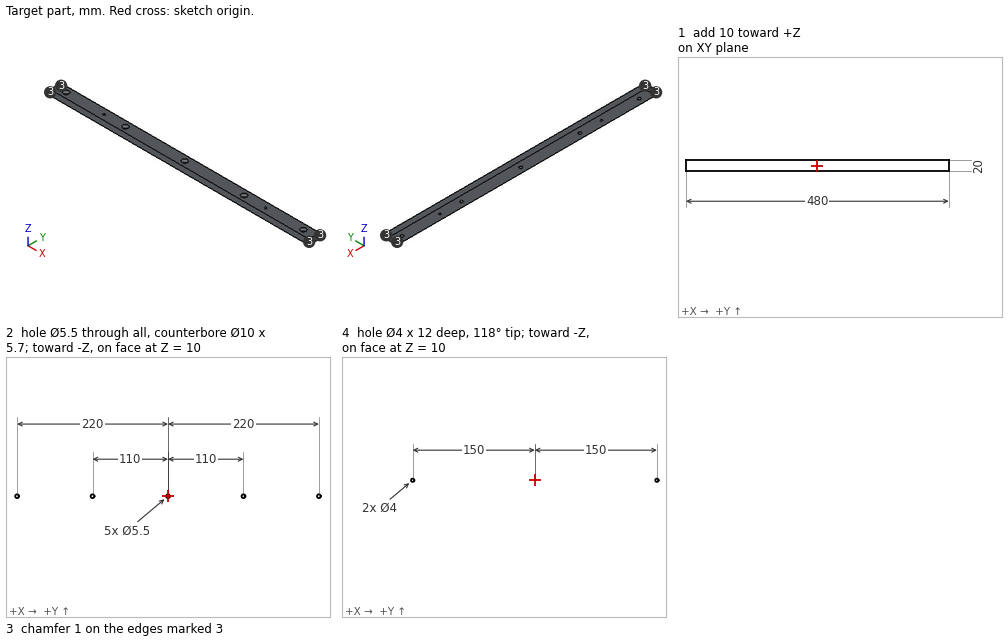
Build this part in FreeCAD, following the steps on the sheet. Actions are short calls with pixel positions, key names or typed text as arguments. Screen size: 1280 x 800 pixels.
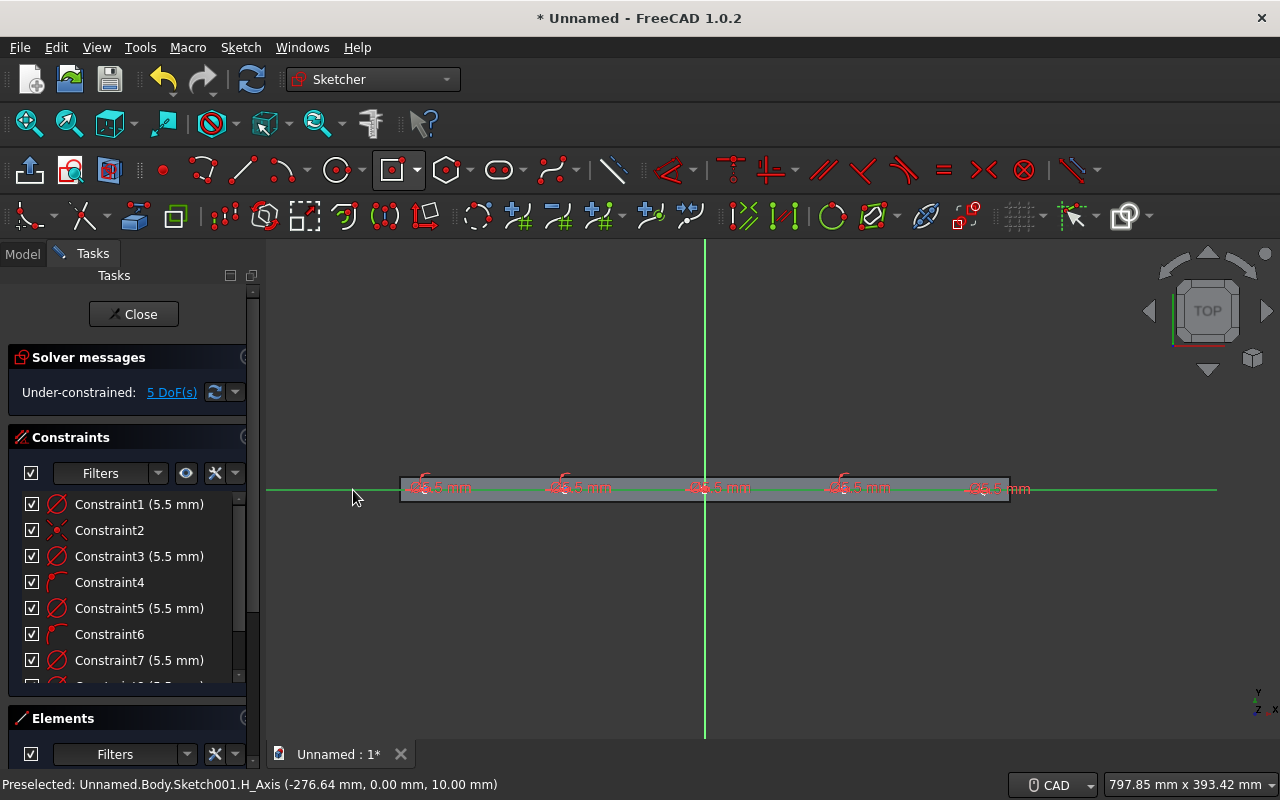
click(732, 170)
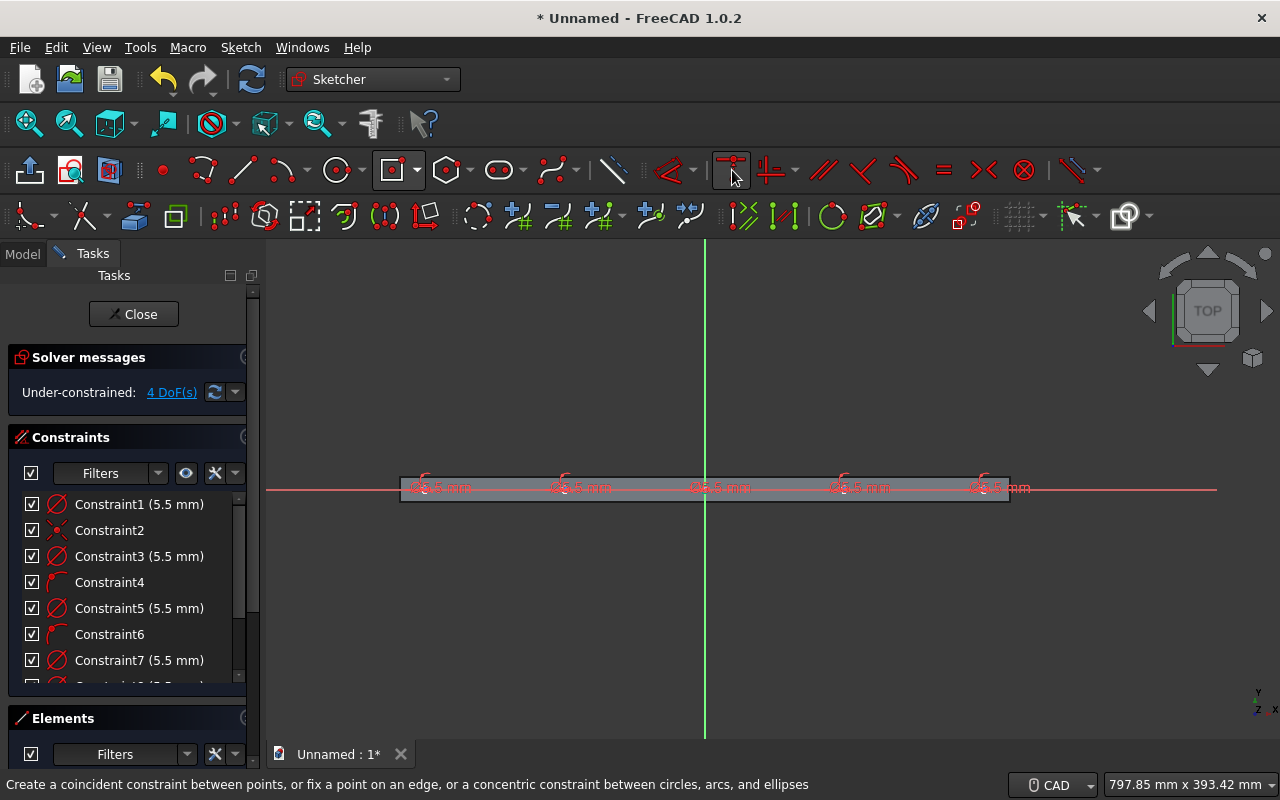
click(668, 170)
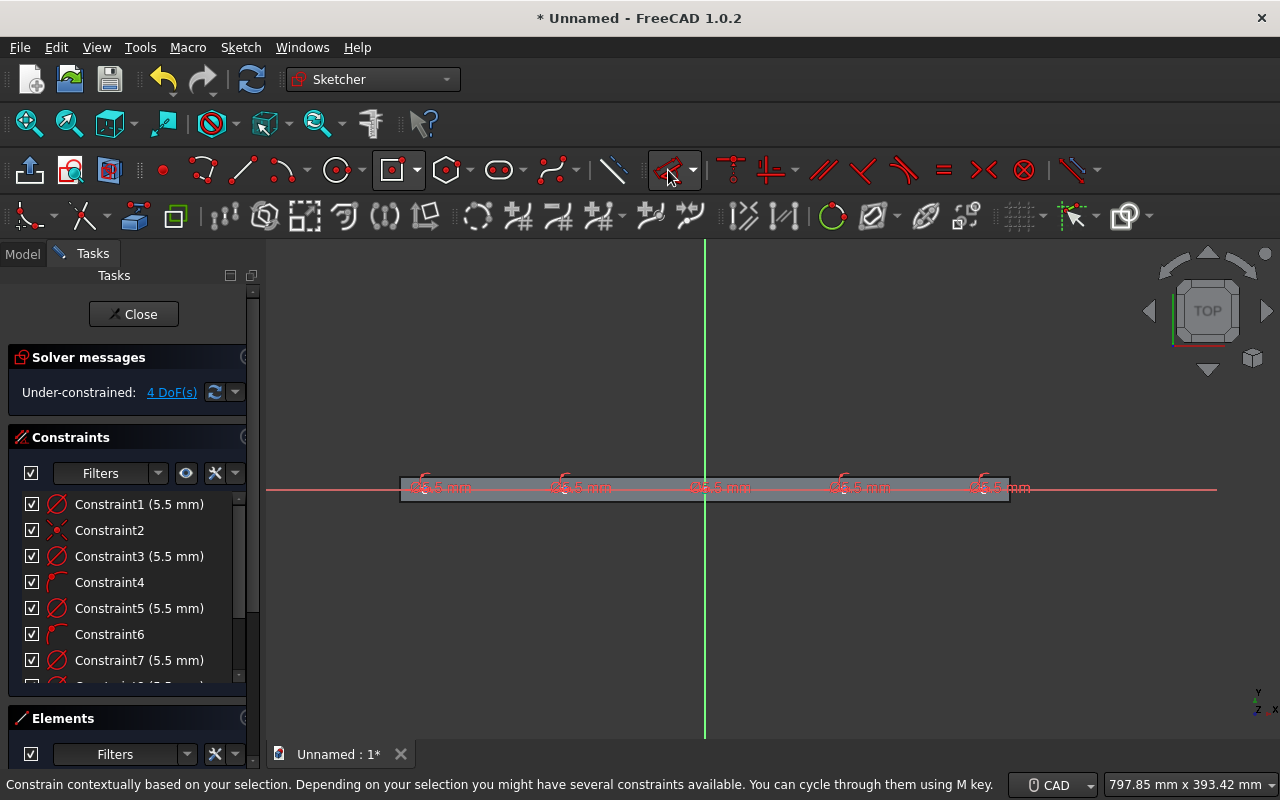
click(565, 490)
click(635, 524)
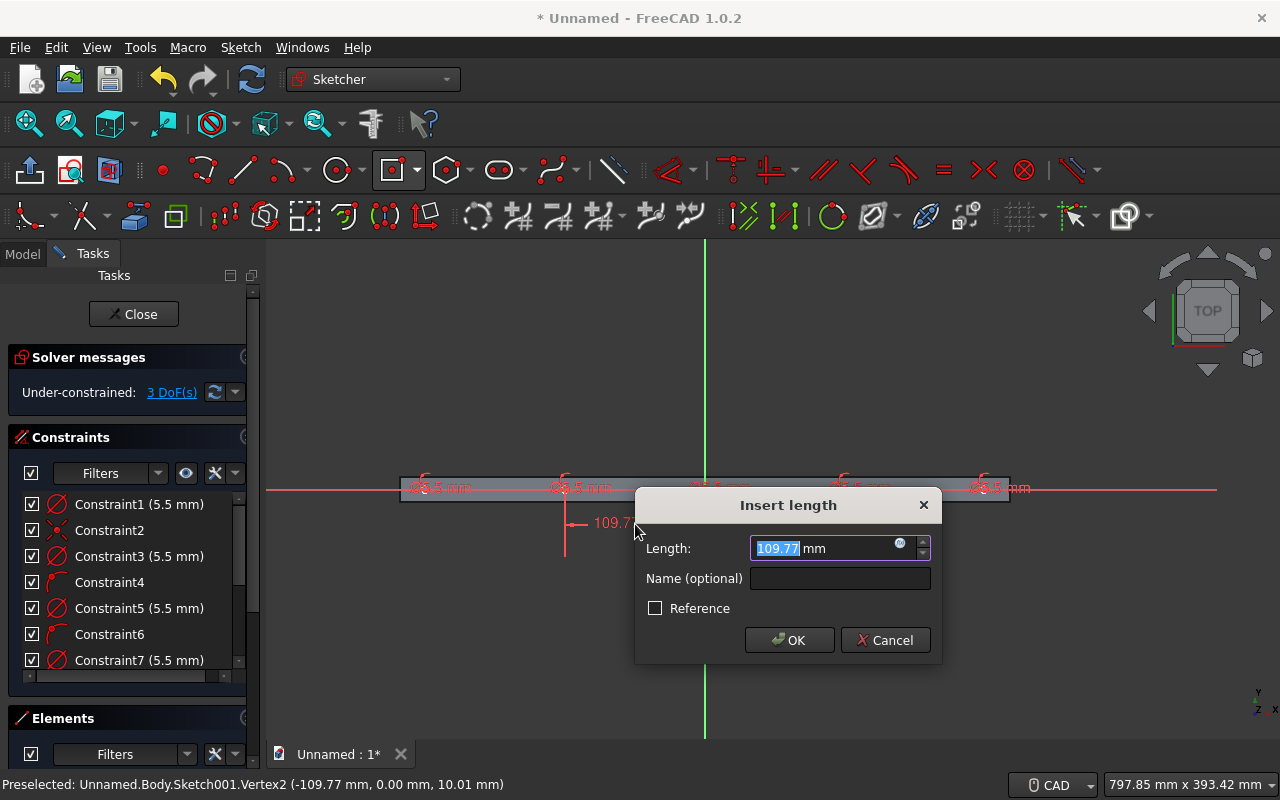
text(110)
key(Return)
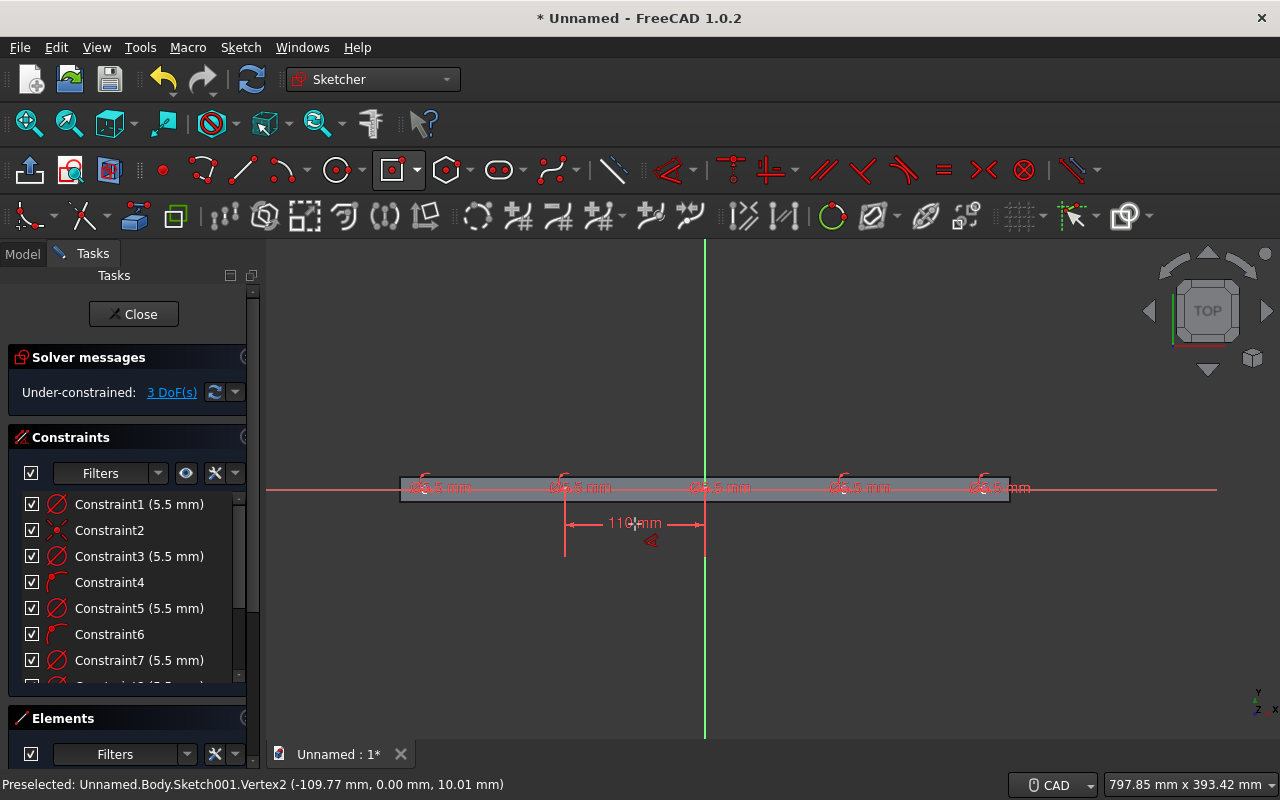
click(844, 490)
click(774, 524)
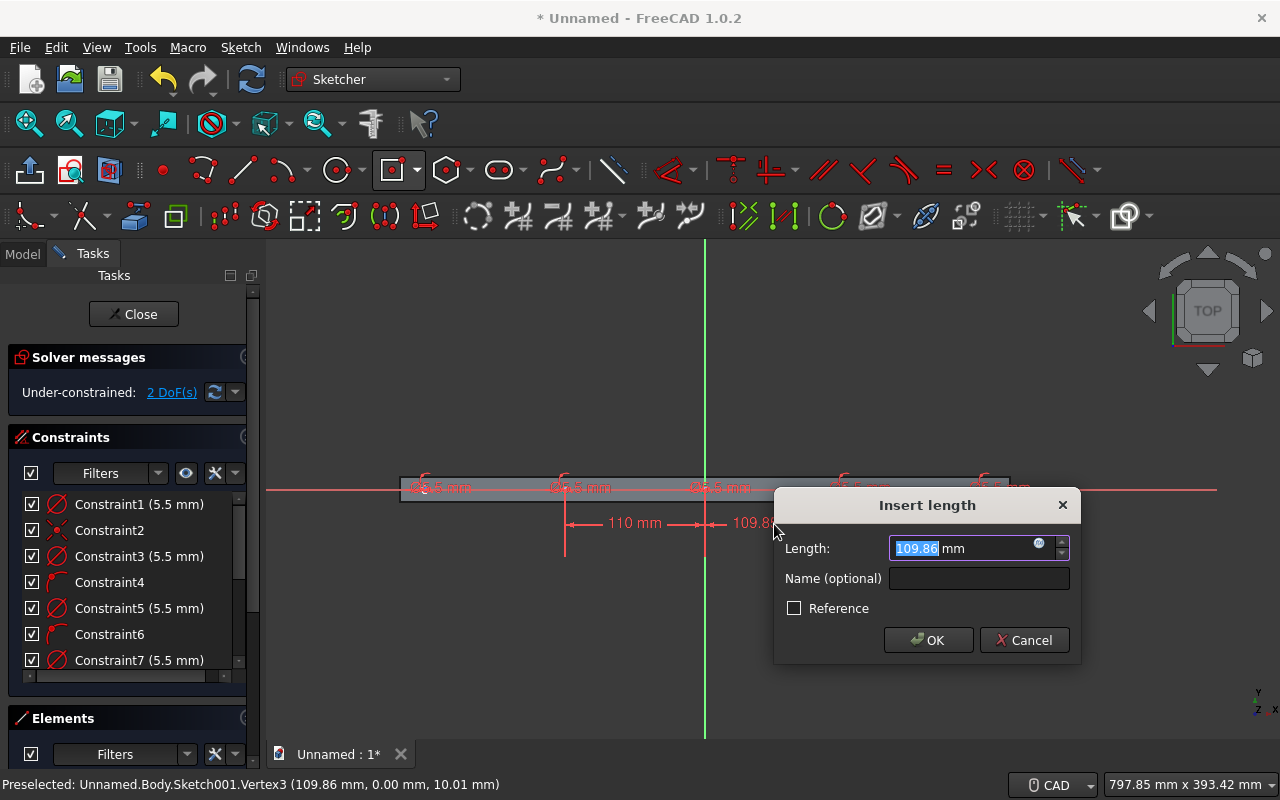
text(110)
key(Return)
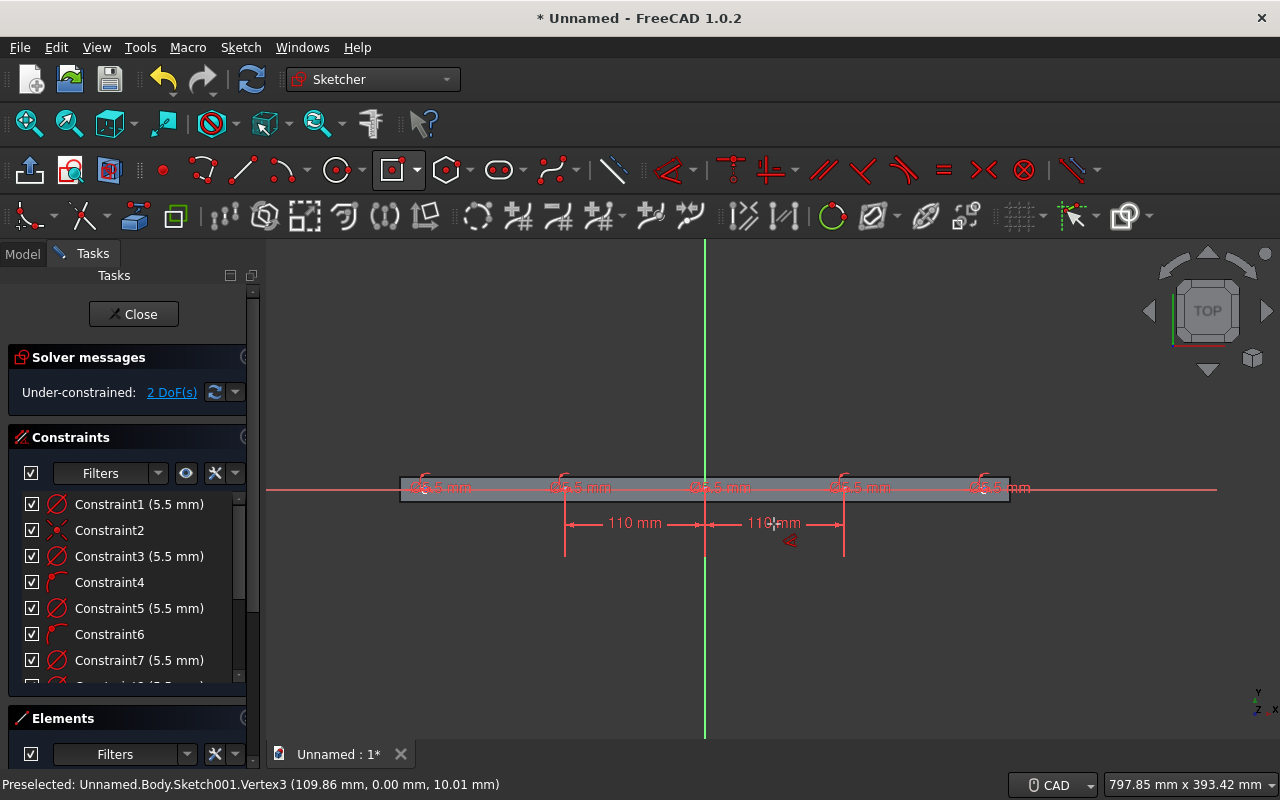
click(984, 490)
click(909, 524)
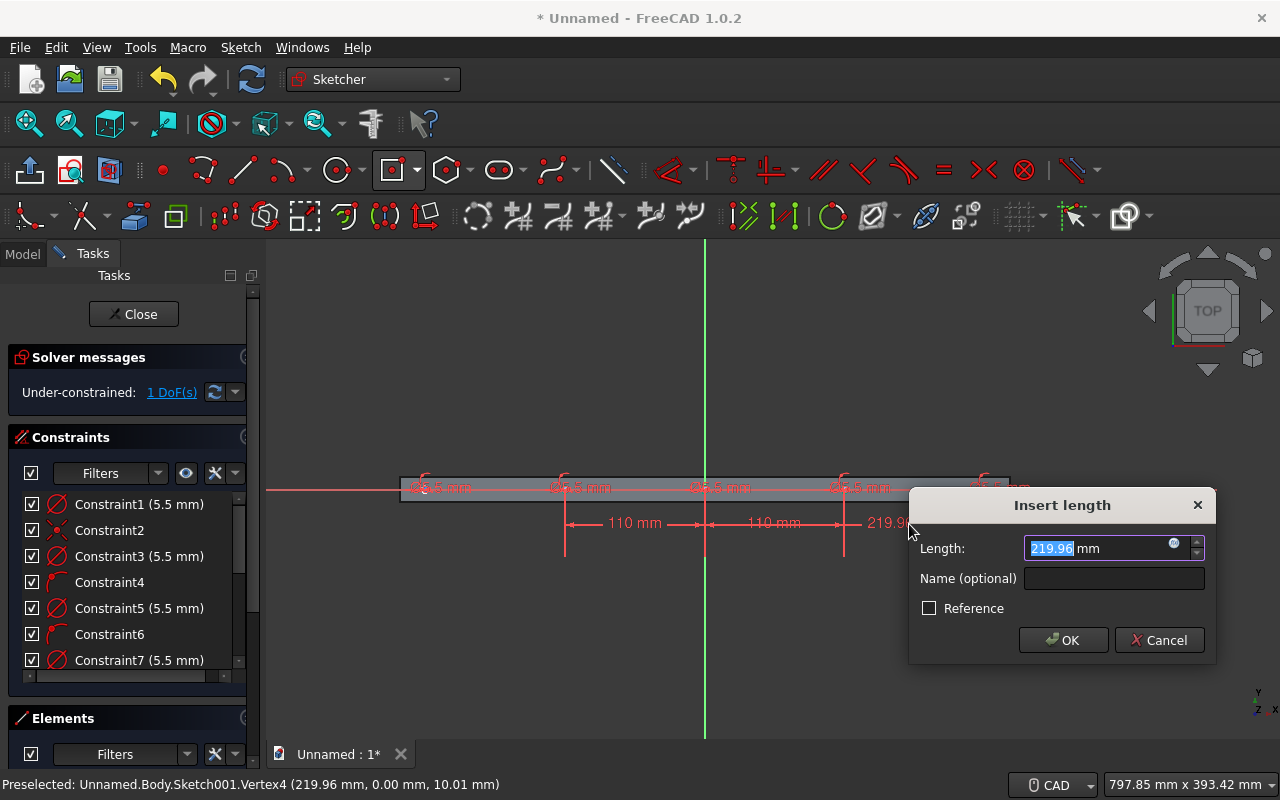
text(220)
key(Return)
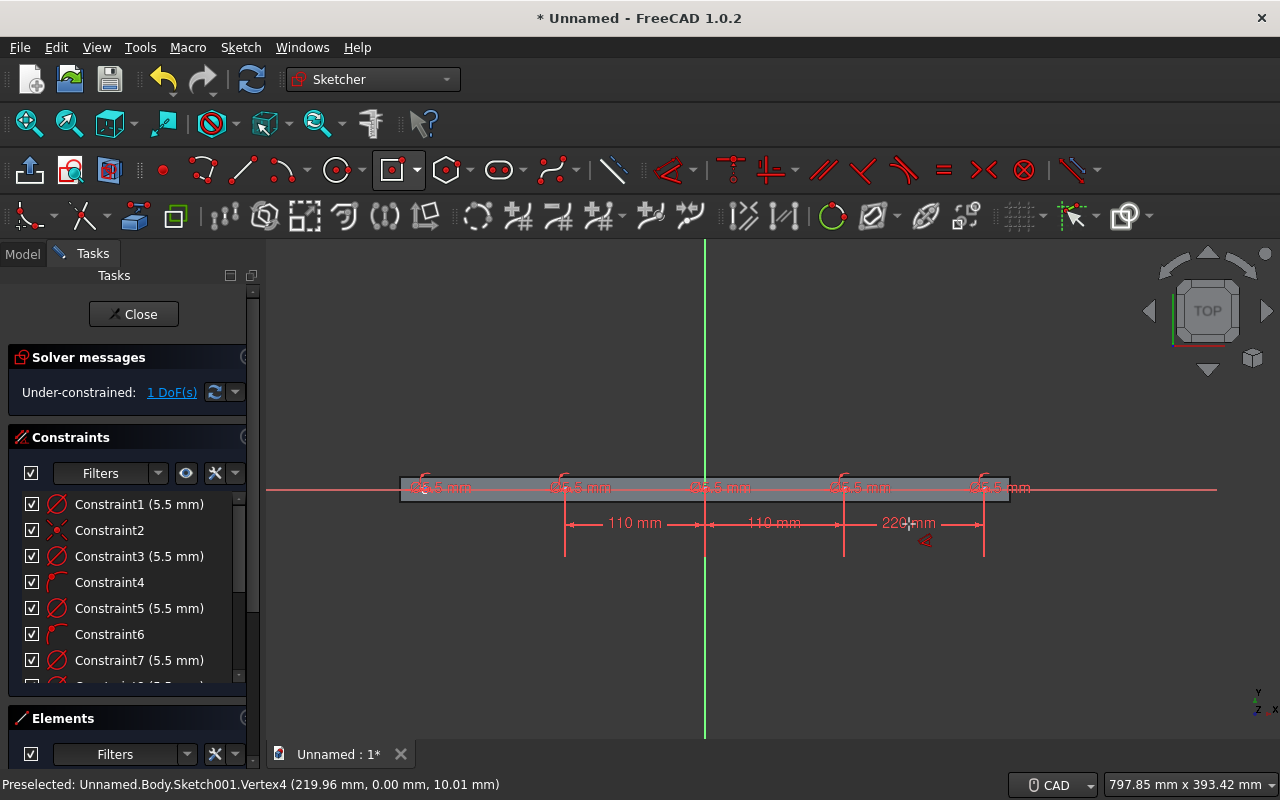
click(425, 490)
click(565, 524)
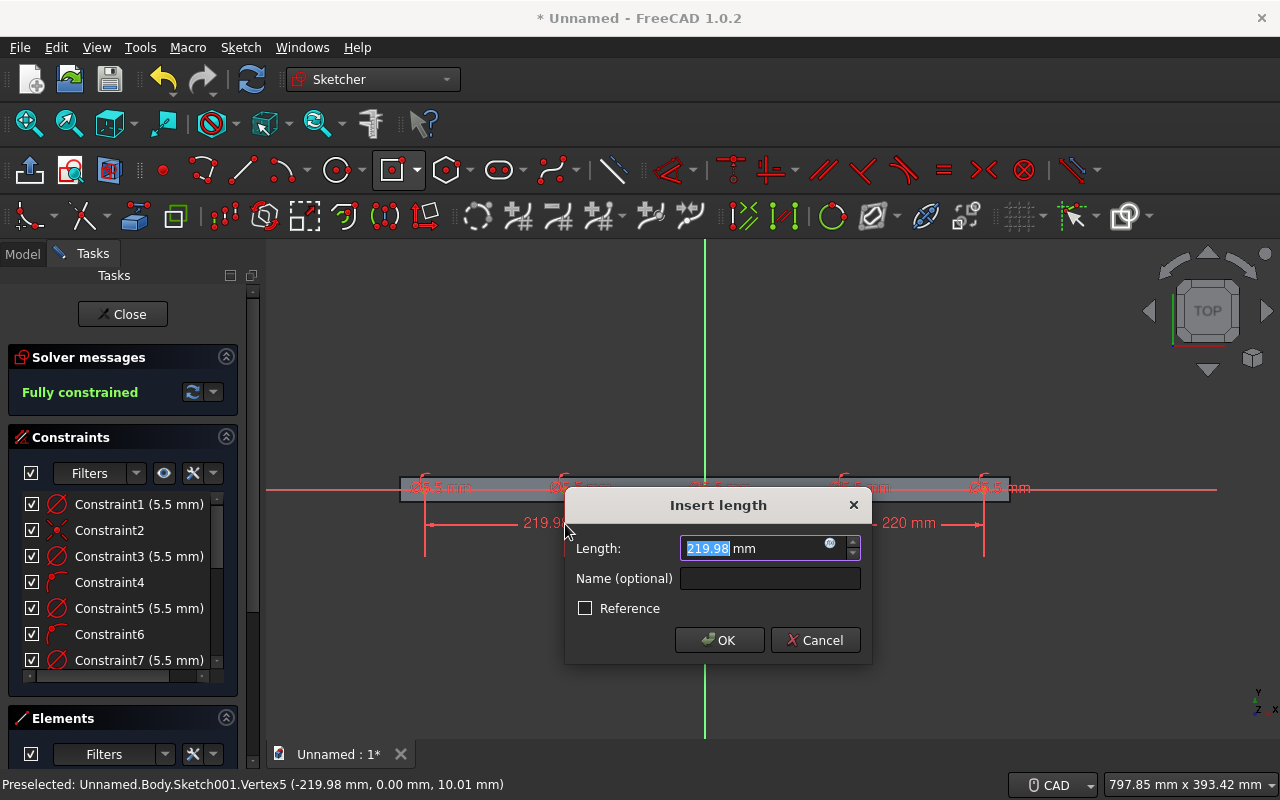
text(220)
key(Return)
key(Escape)